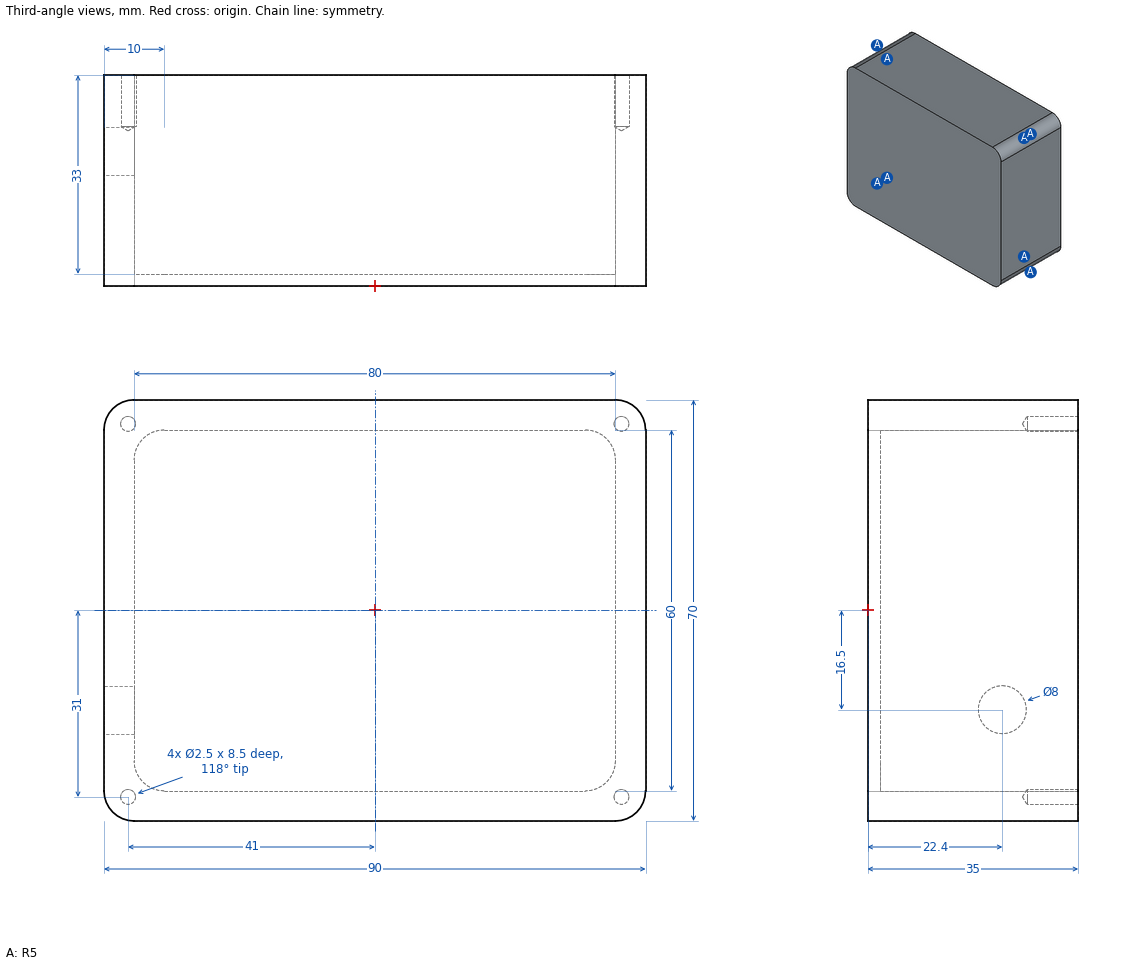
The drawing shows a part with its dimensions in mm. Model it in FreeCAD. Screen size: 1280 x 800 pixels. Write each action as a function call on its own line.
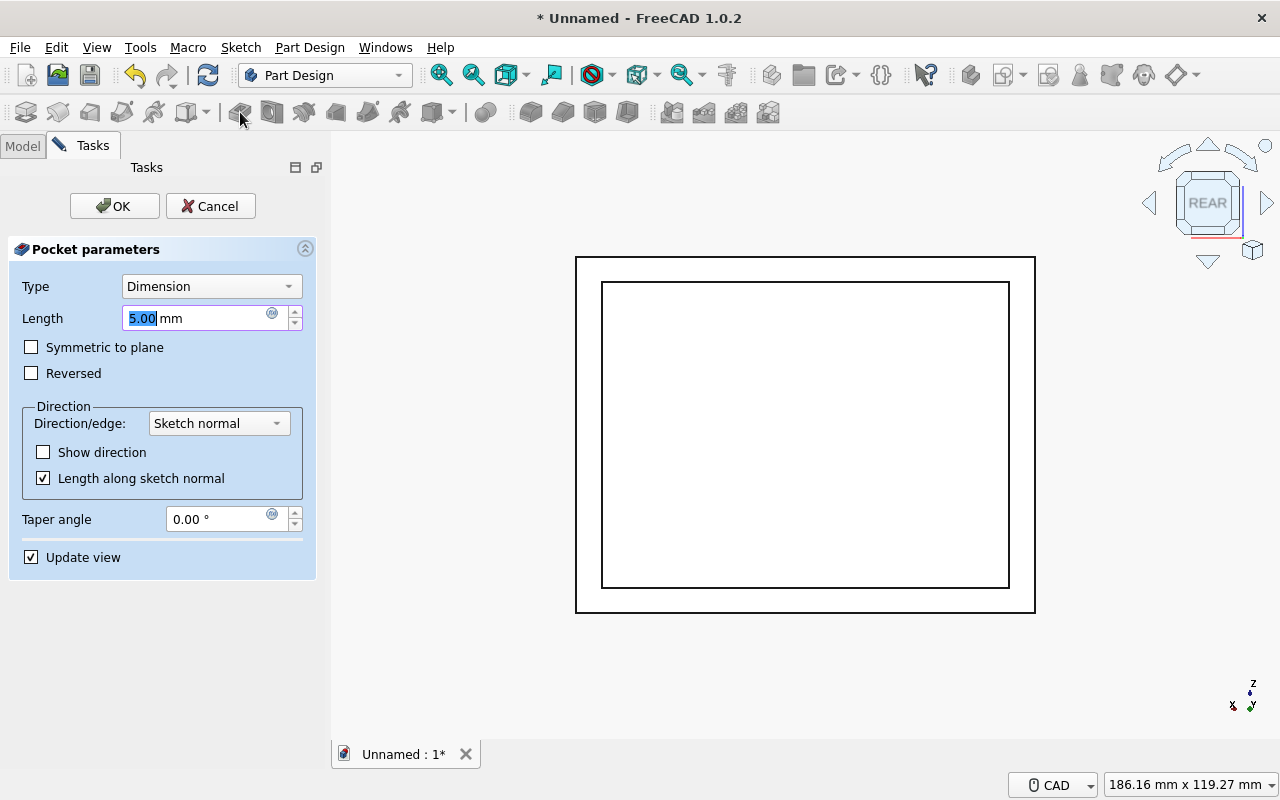
text(33)
key(Tab)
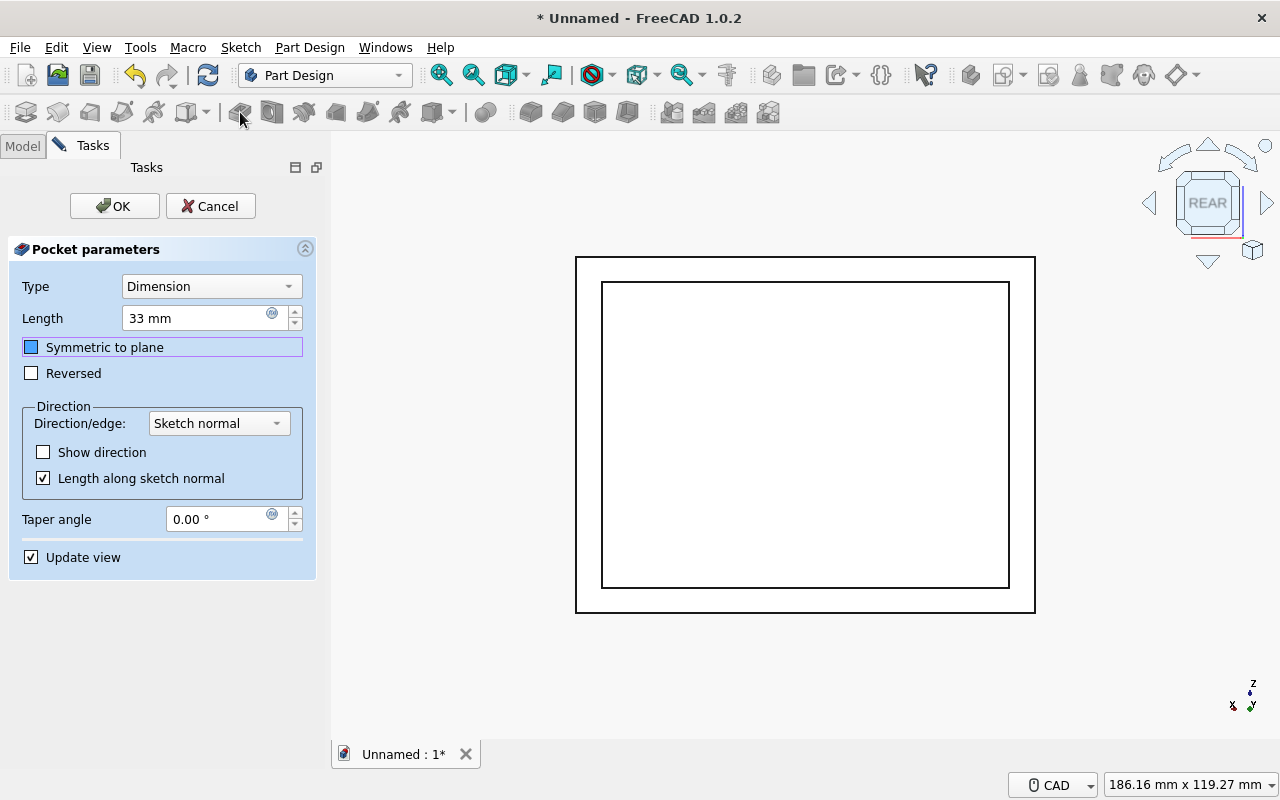
click(115, 206)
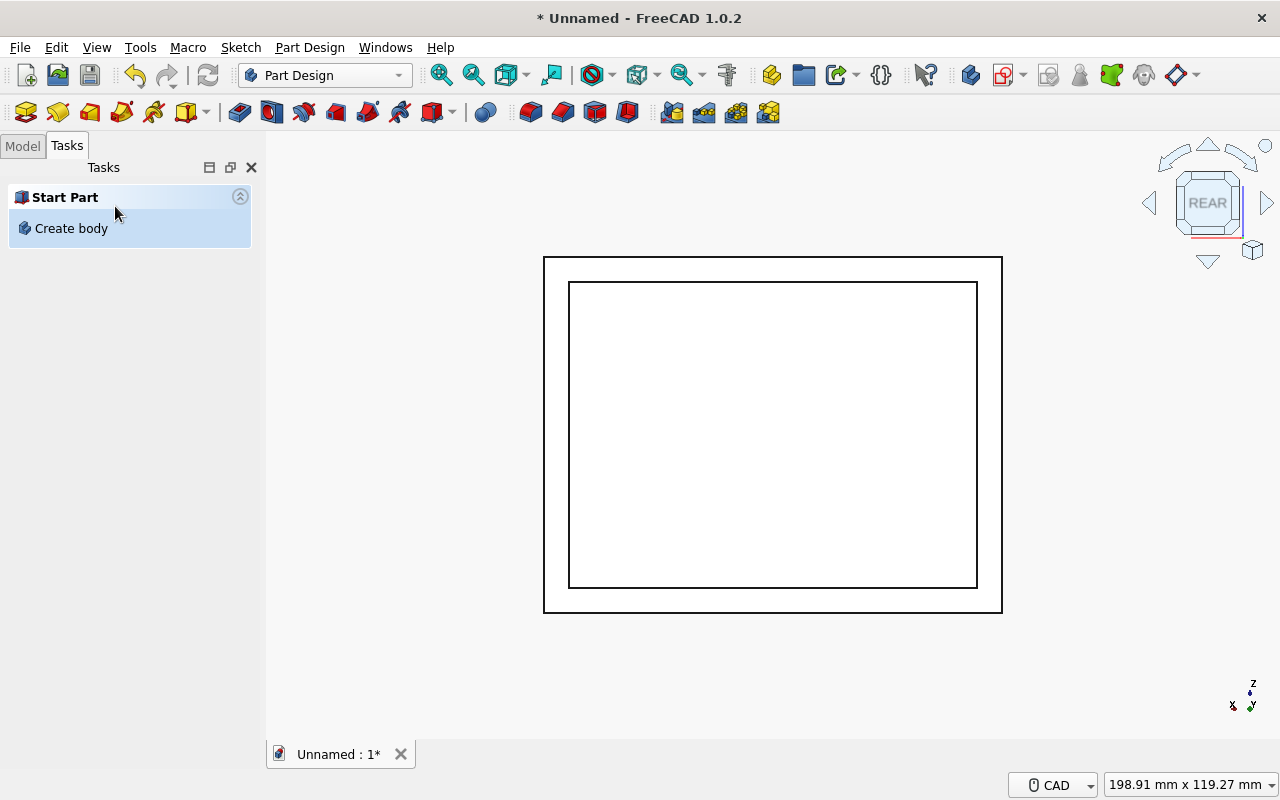
key(0)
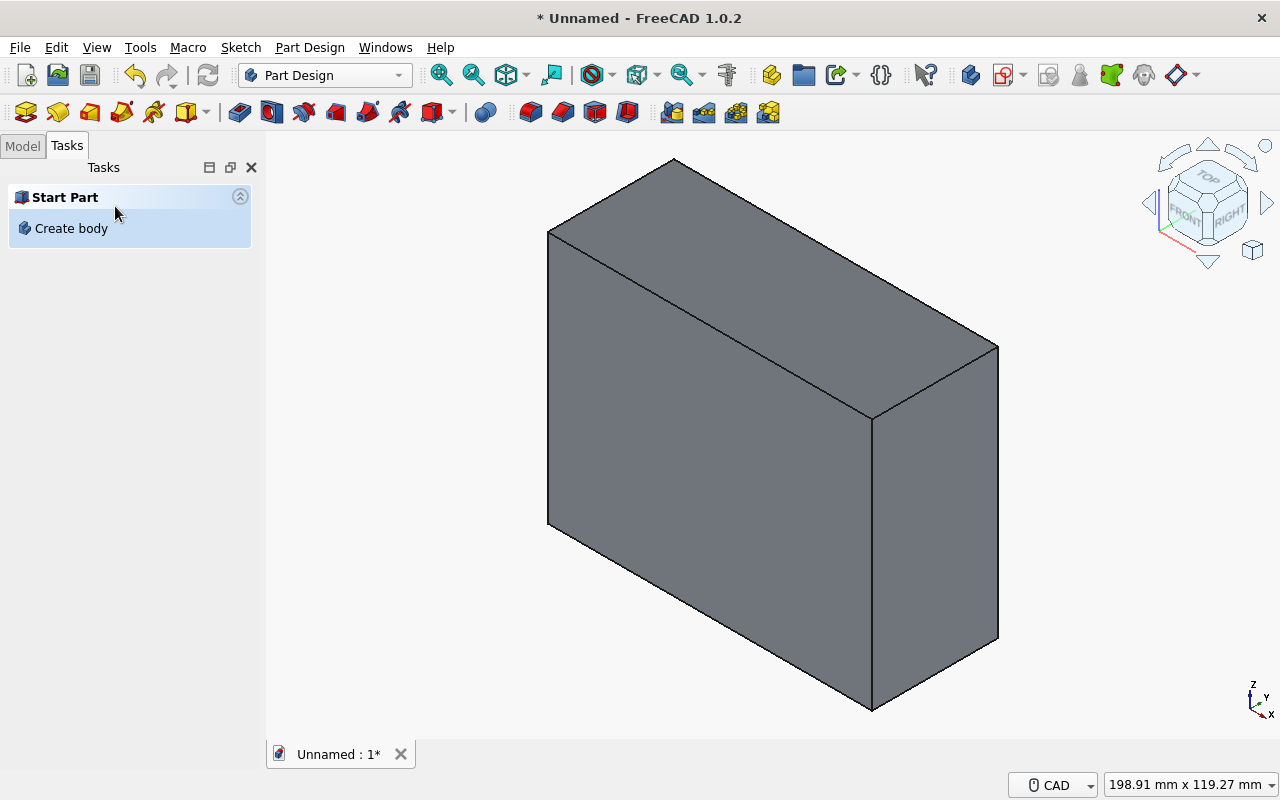
click(935, 382)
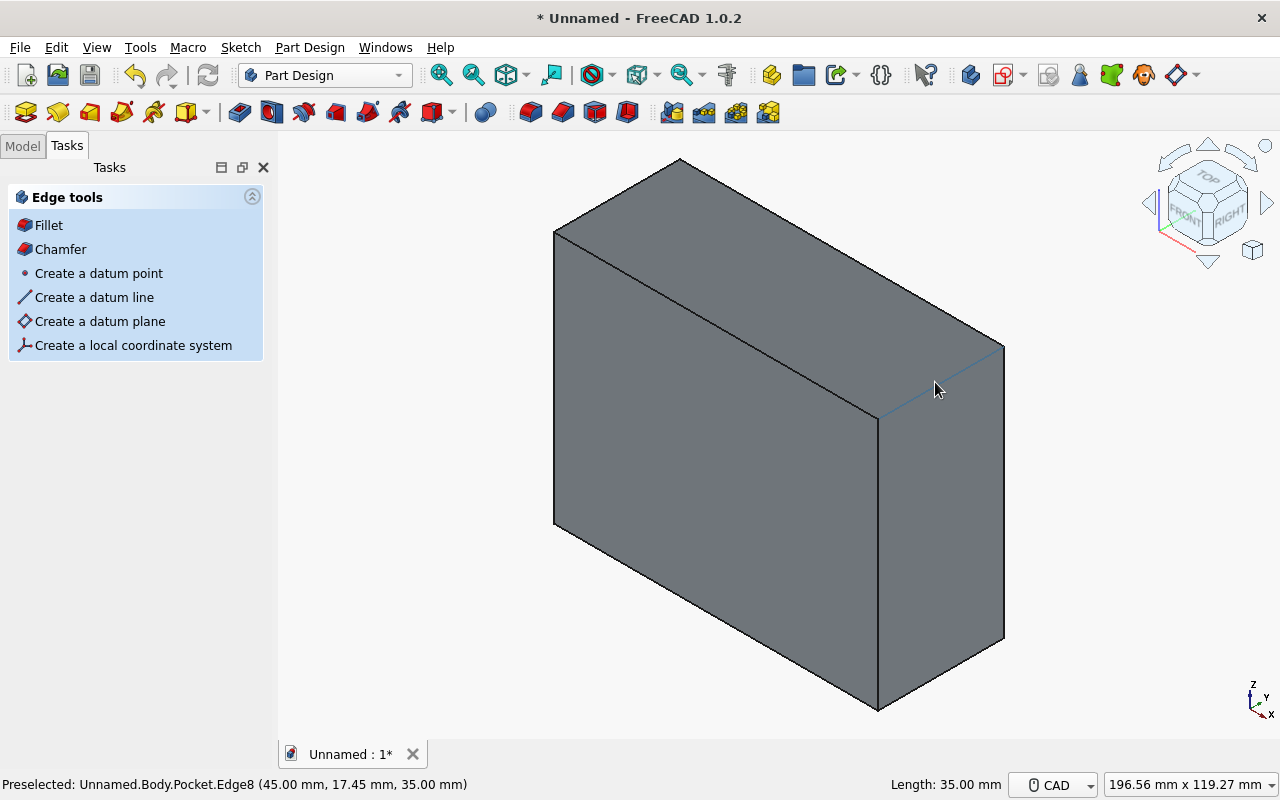
key(2)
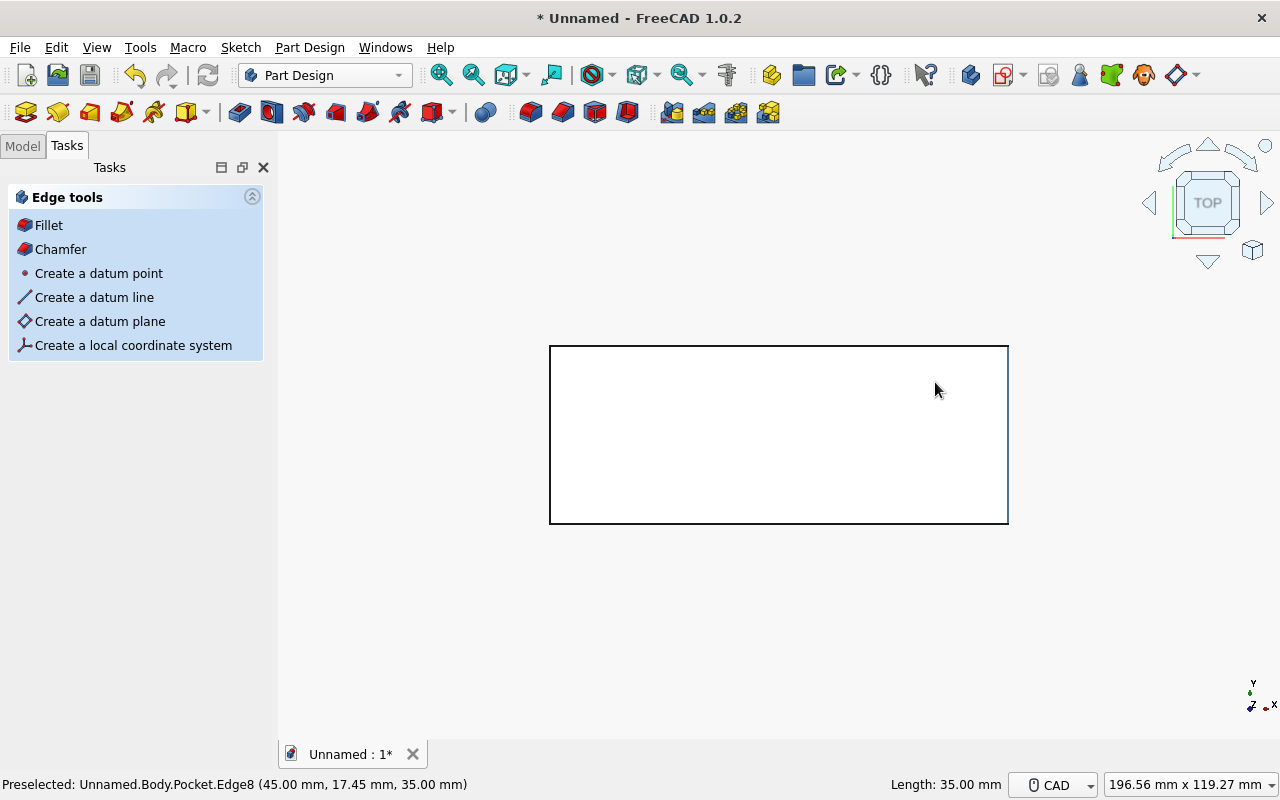
click(550, 434, ctrl)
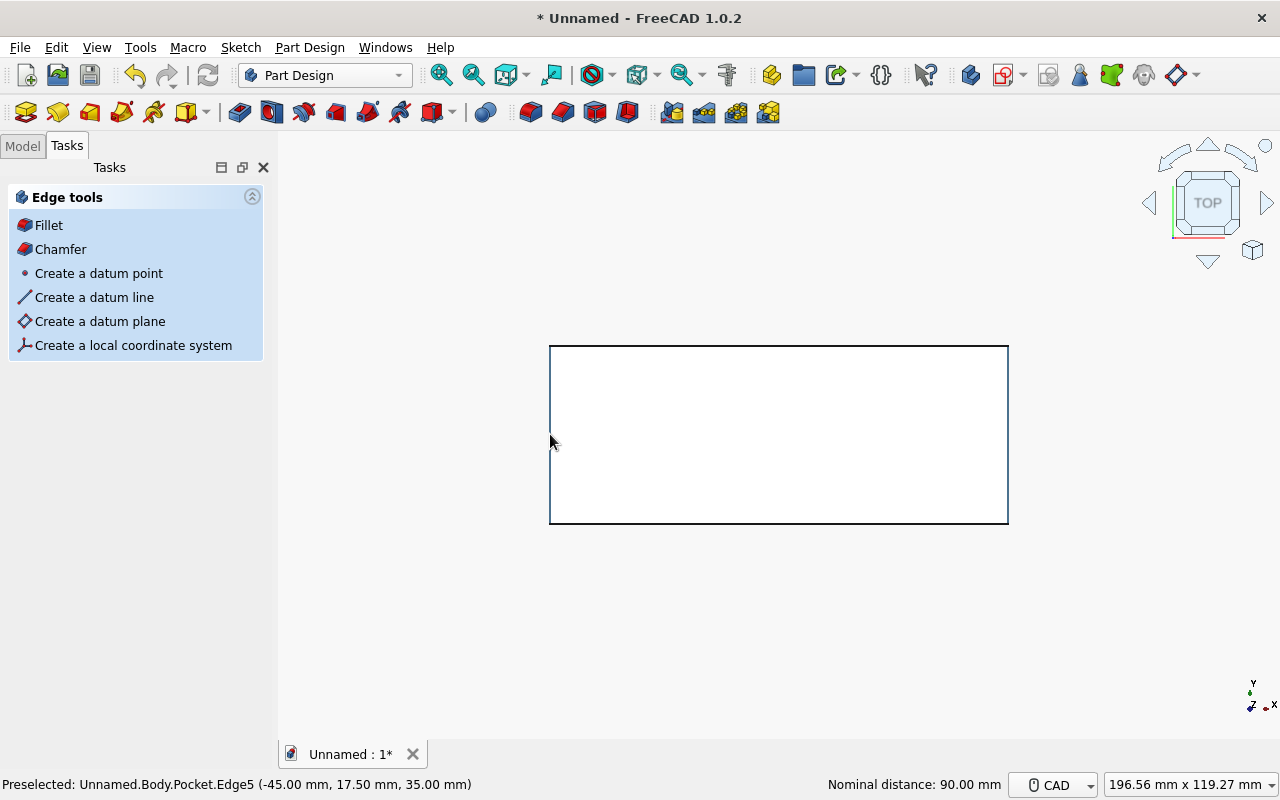
key(1)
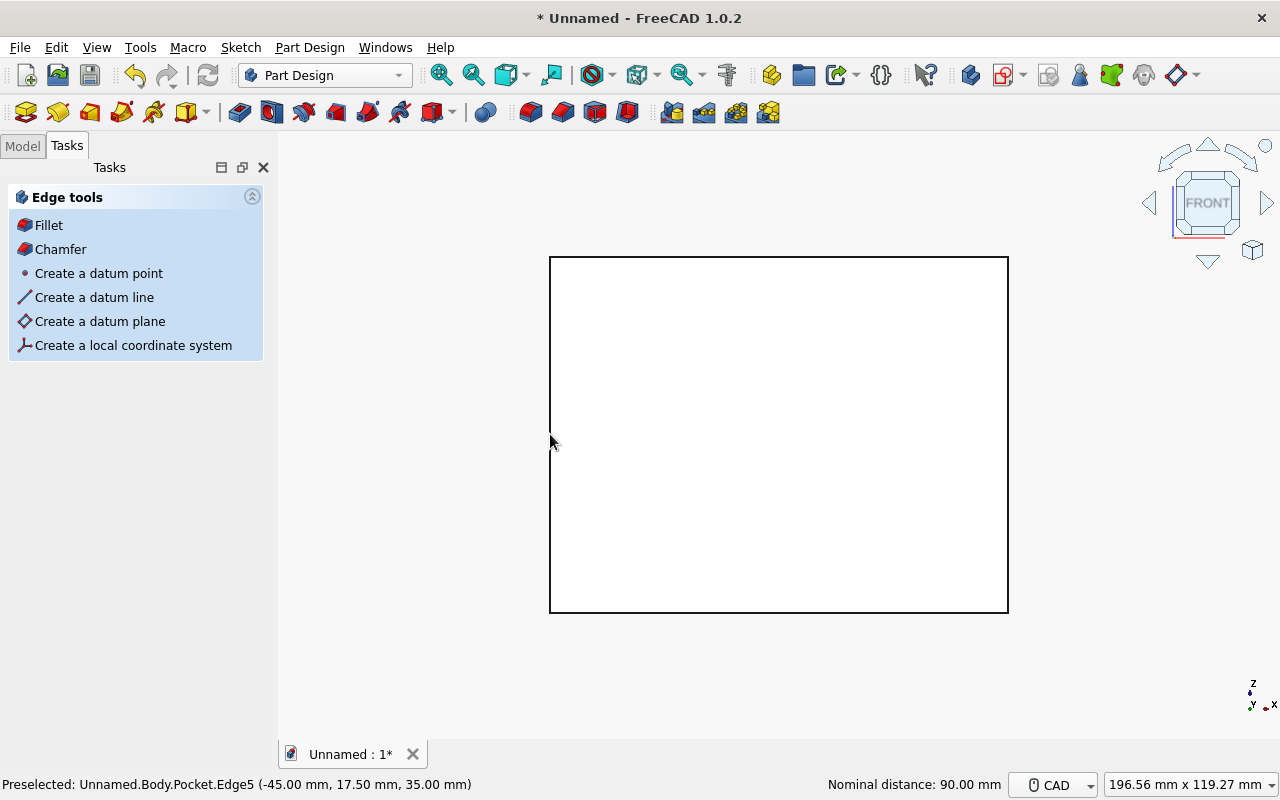
key(3)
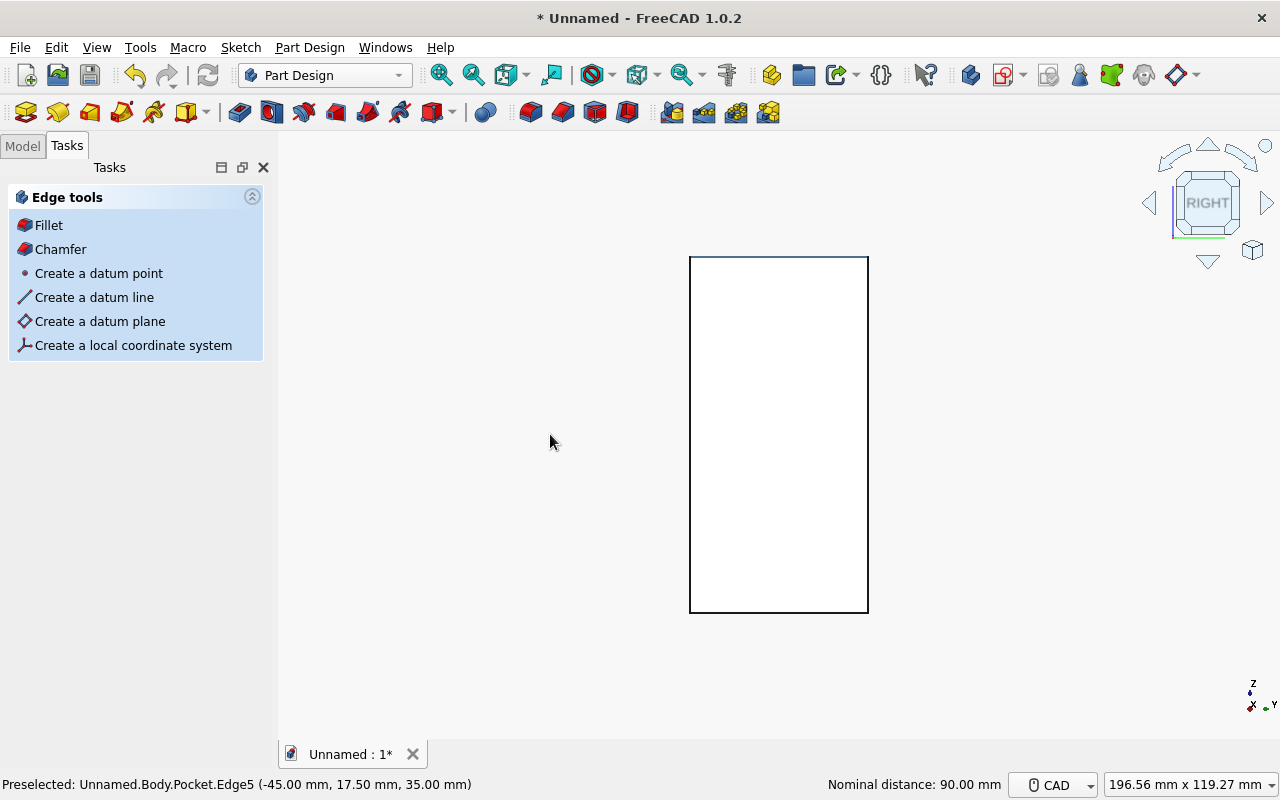
click(779, 612, ctrl)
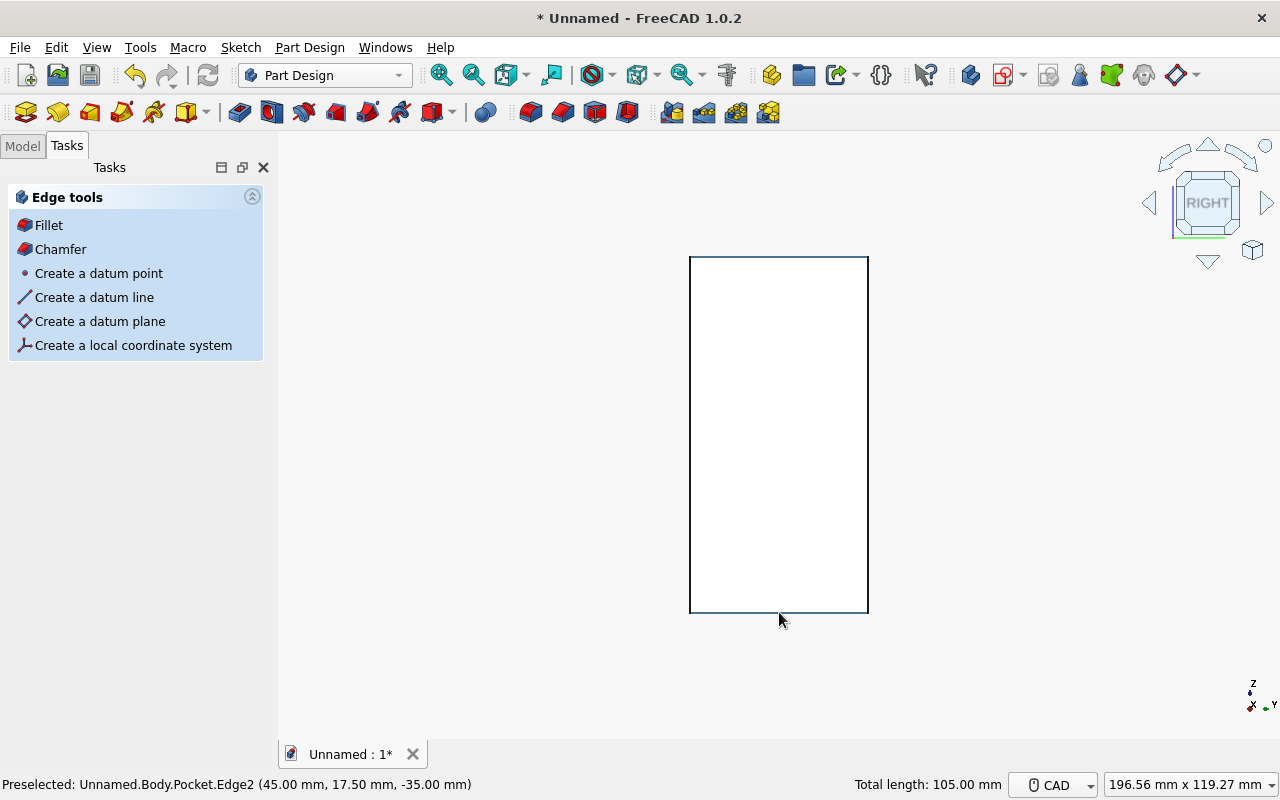
key(5)